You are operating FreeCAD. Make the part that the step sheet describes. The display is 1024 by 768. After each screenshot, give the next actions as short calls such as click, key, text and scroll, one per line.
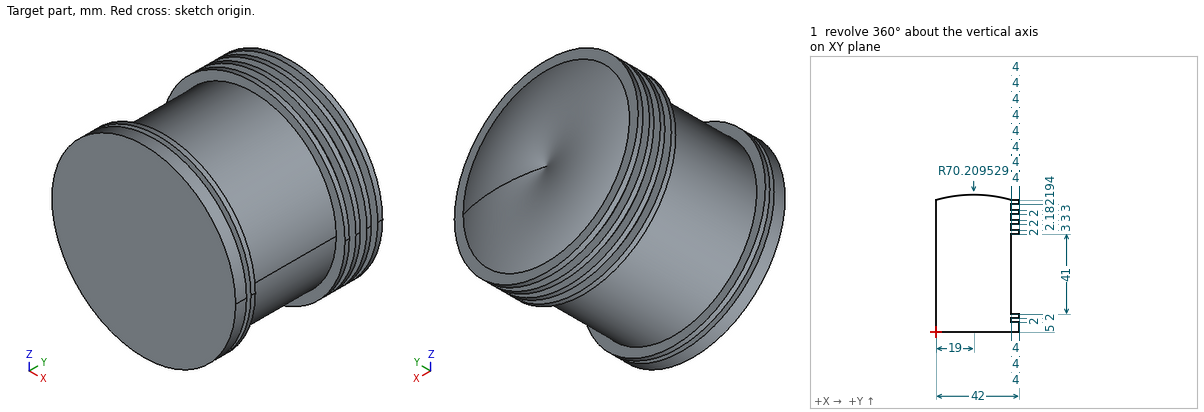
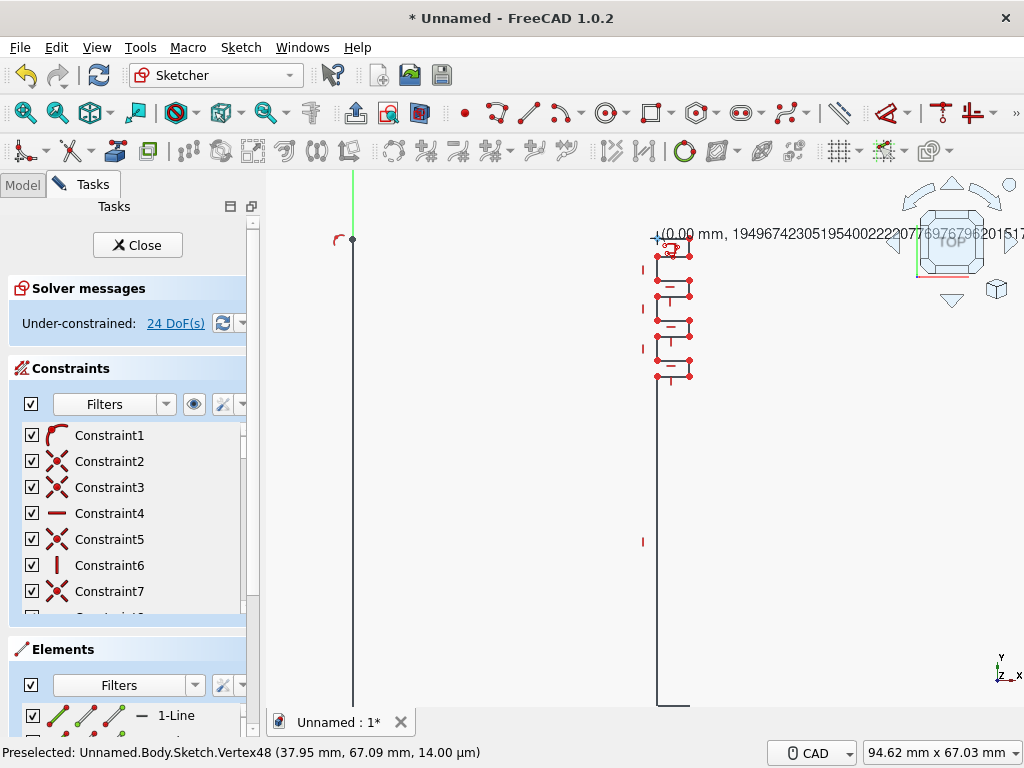
key(g)
key(3)
key(a)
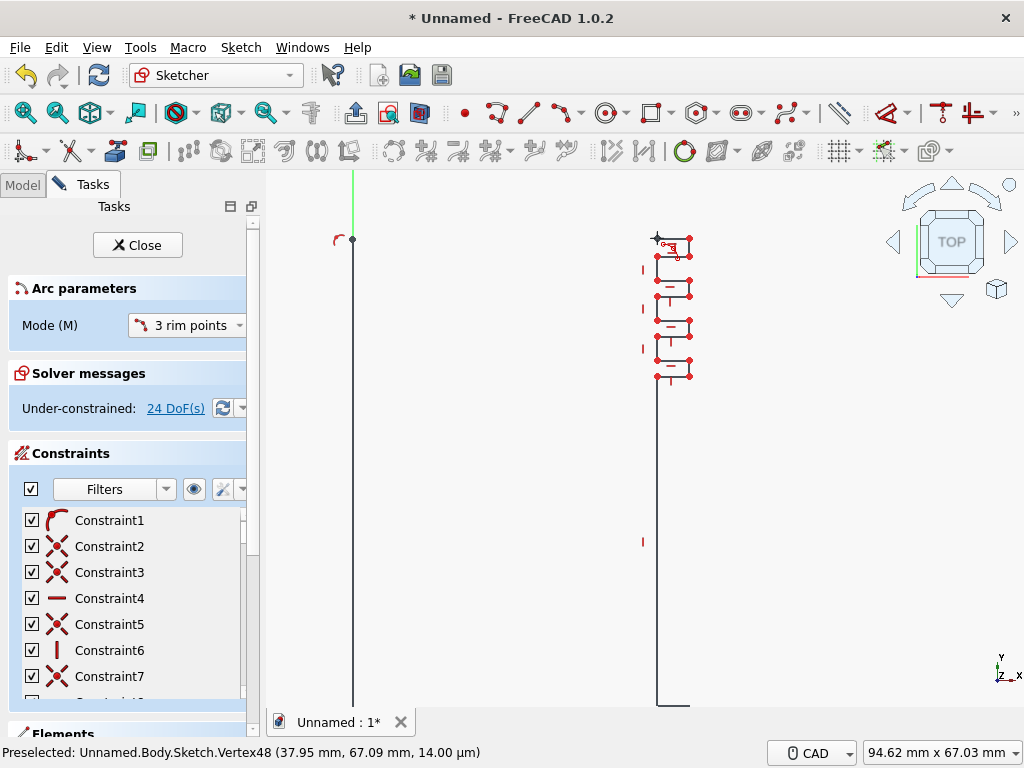
click(657, 239)
click(353, 240)
click(505, 217)
key(Escape)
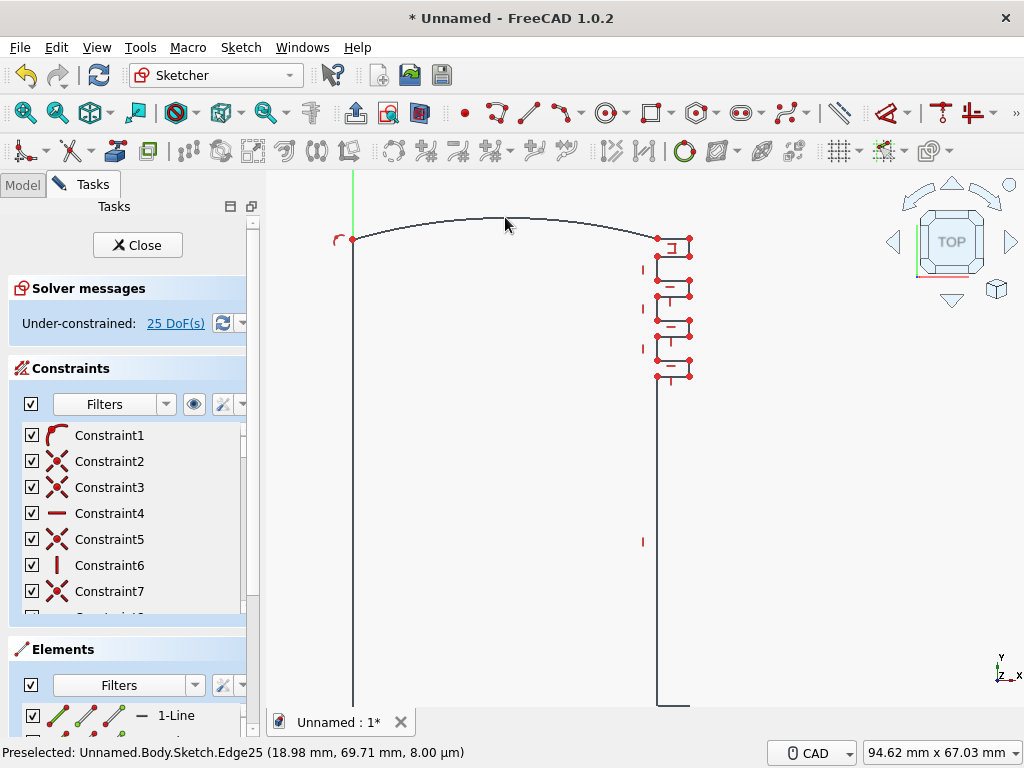
key(d)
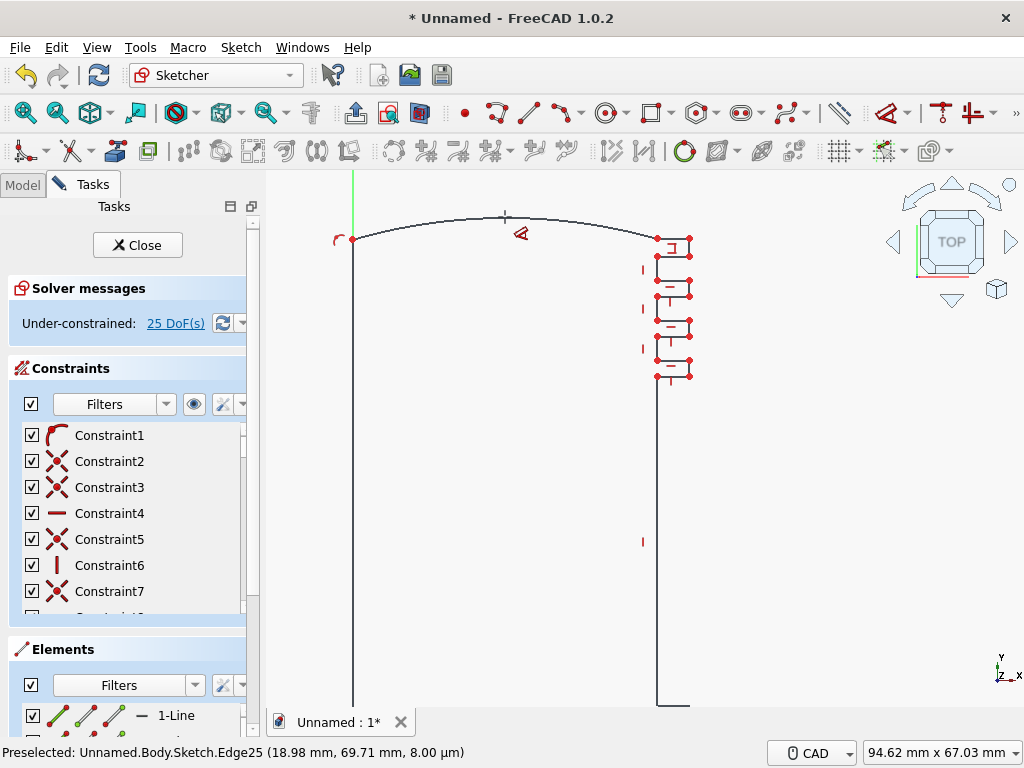
click(566, 221)
click(840, 290)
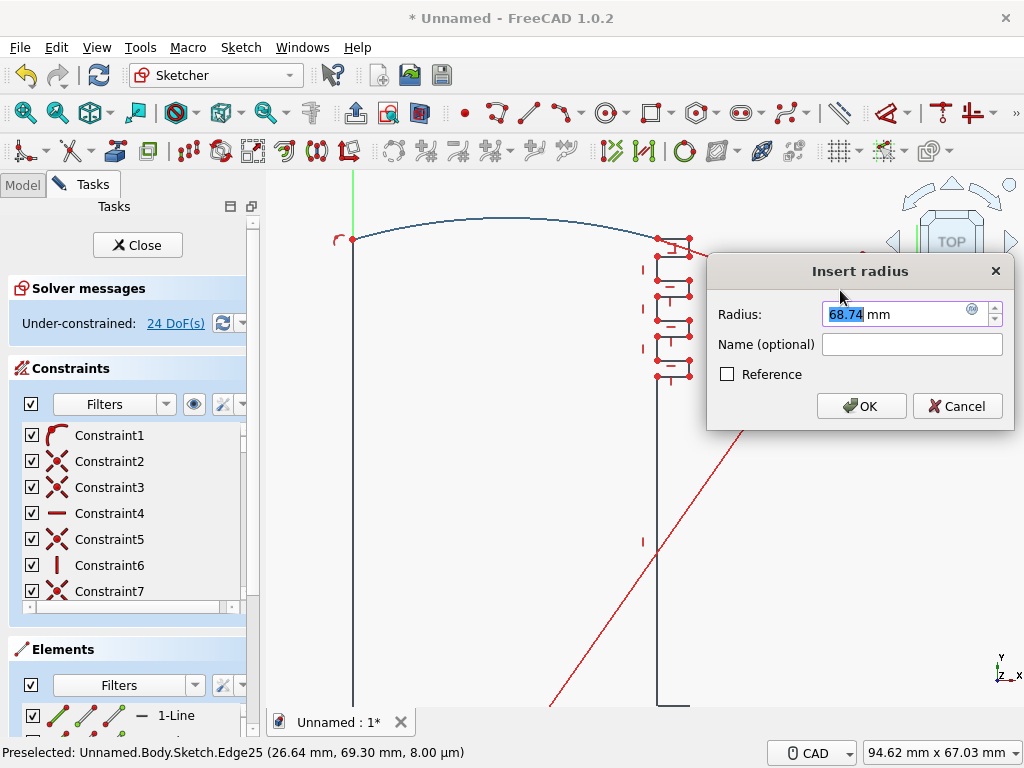
text(70.209529)
key(Return)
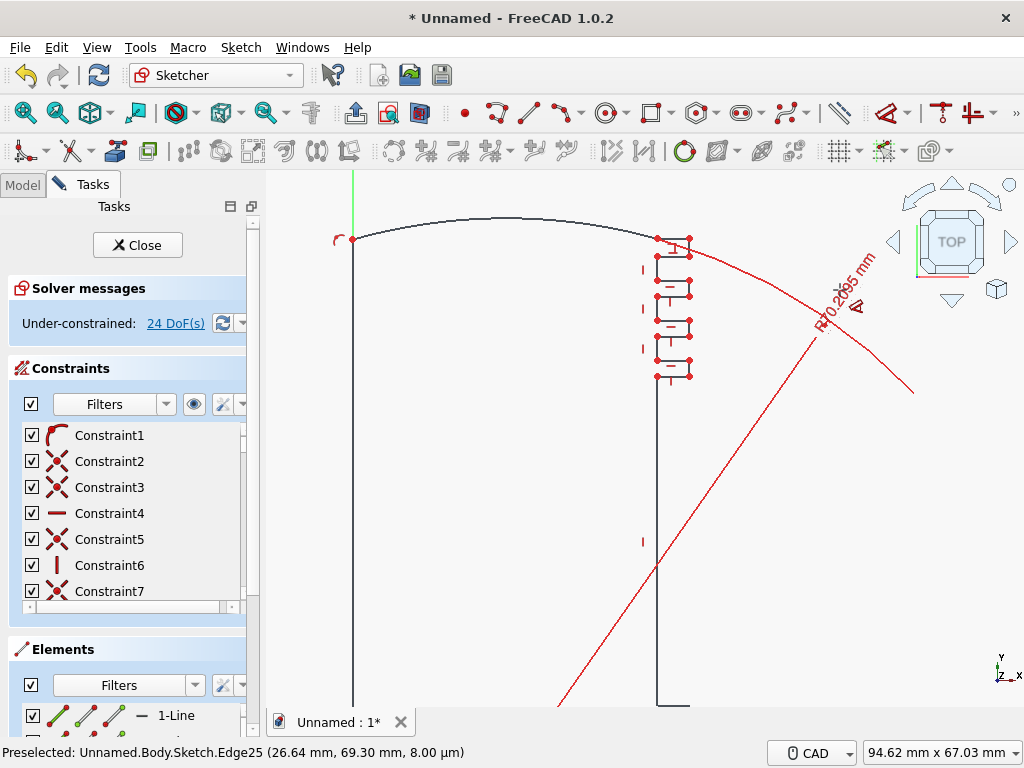
scroll(689, 320, down, 2)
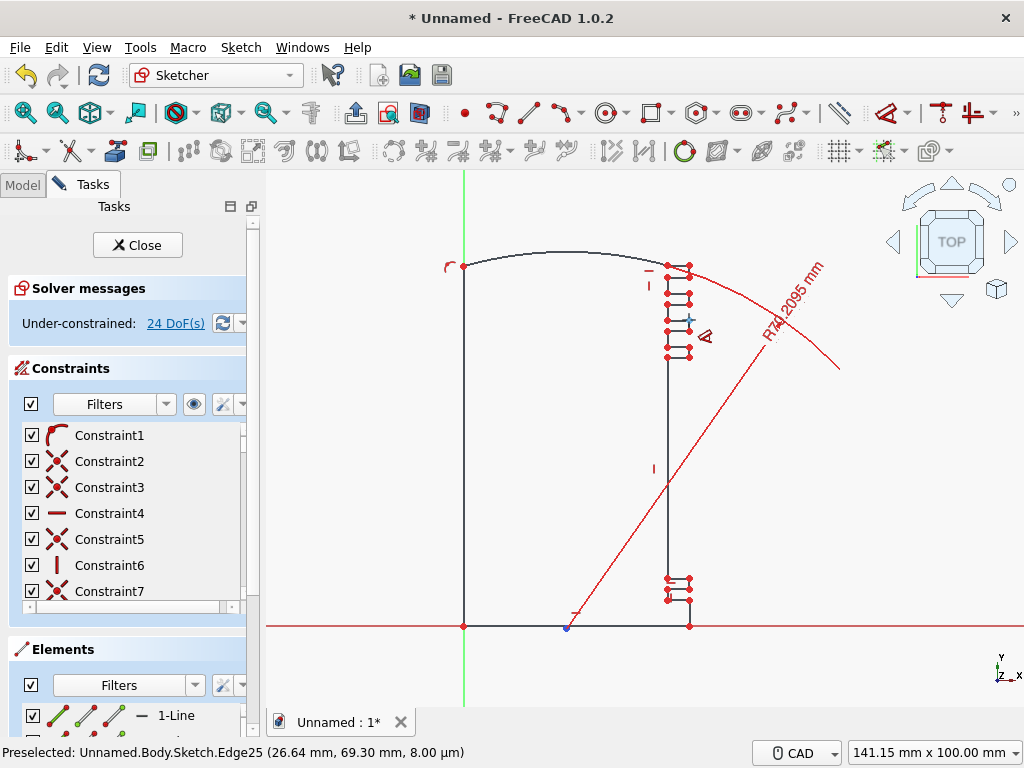
scroll(690, 618, up, 3)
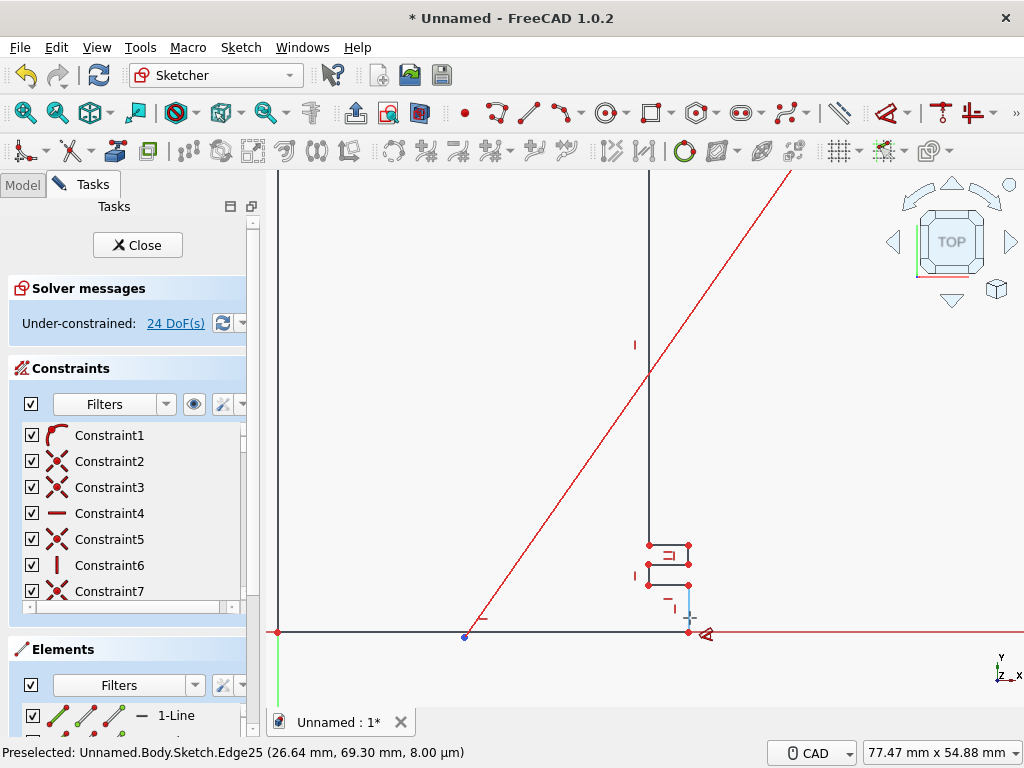
click(689, 618)
click(723, 609)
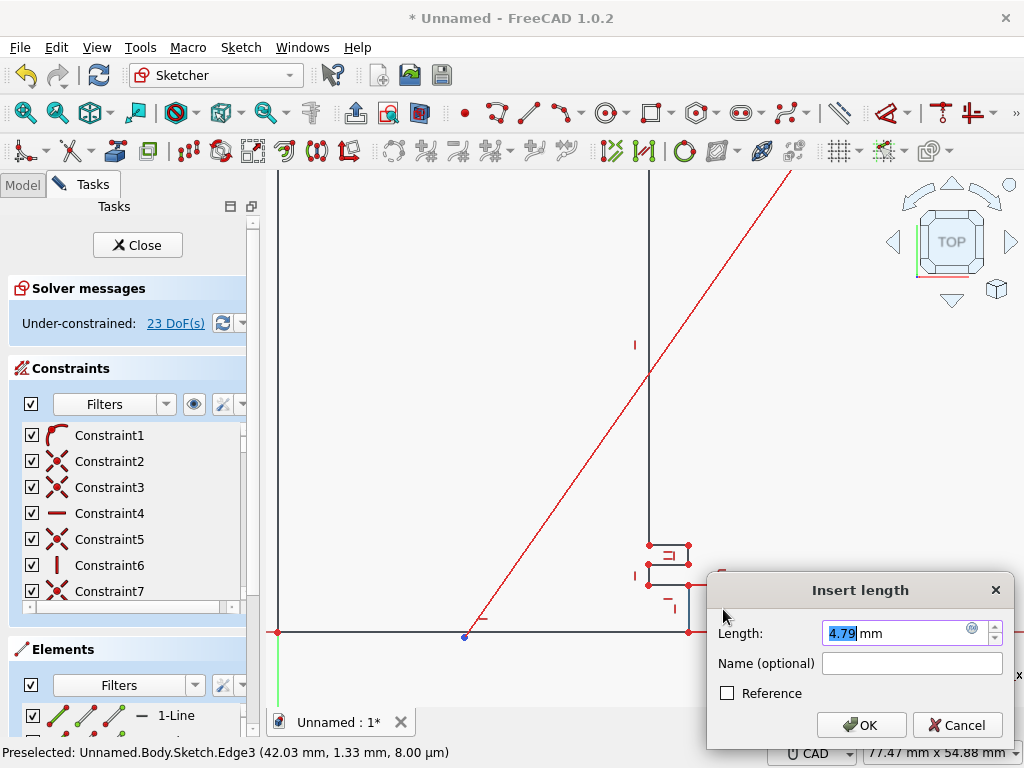
text(5)
key(Return)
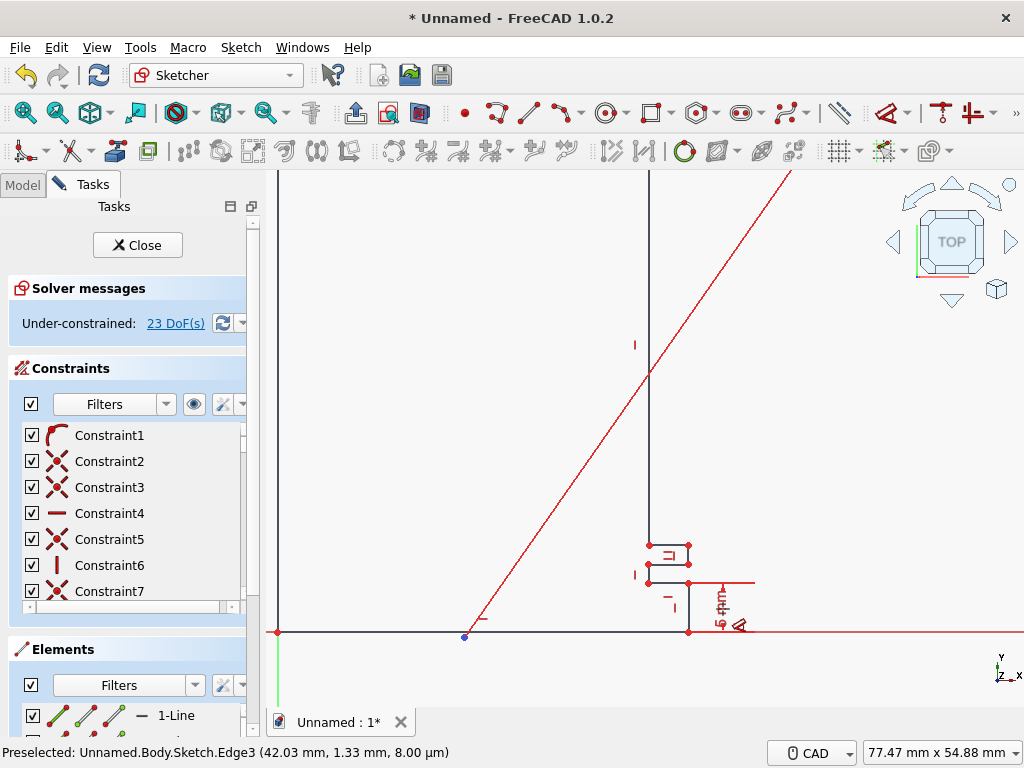
click(677, 583)
click(669, 525)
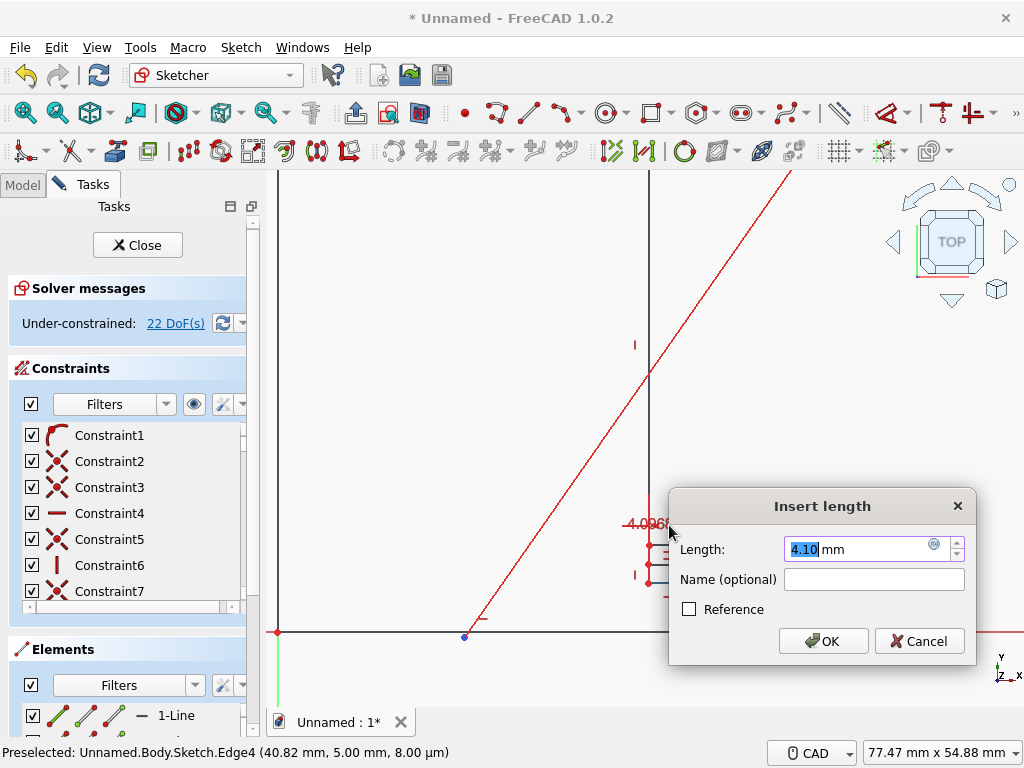
text(4)
key(Return)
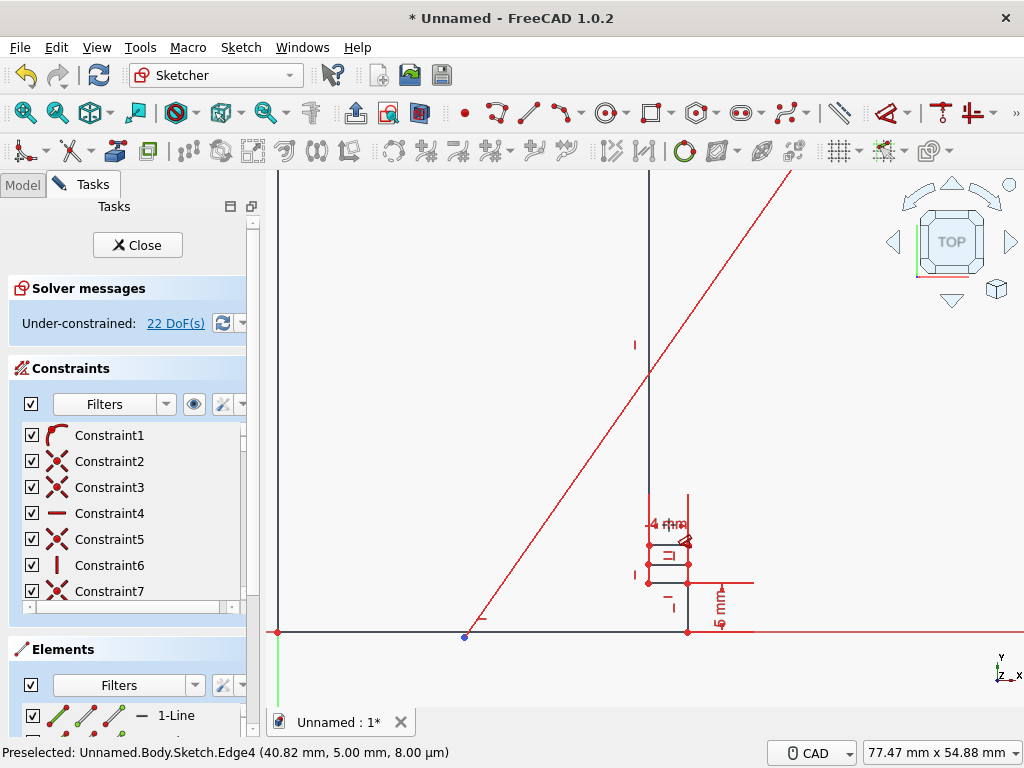
scroll(649, 574, up, 4)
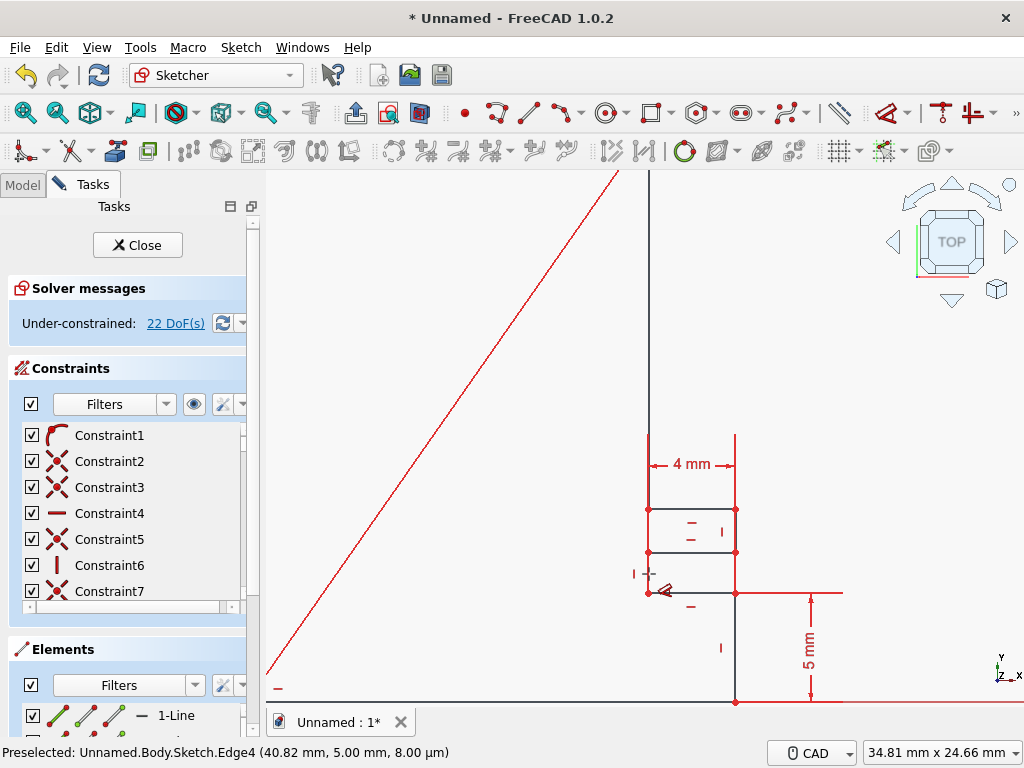
click(648, 573)
click(682, 573)